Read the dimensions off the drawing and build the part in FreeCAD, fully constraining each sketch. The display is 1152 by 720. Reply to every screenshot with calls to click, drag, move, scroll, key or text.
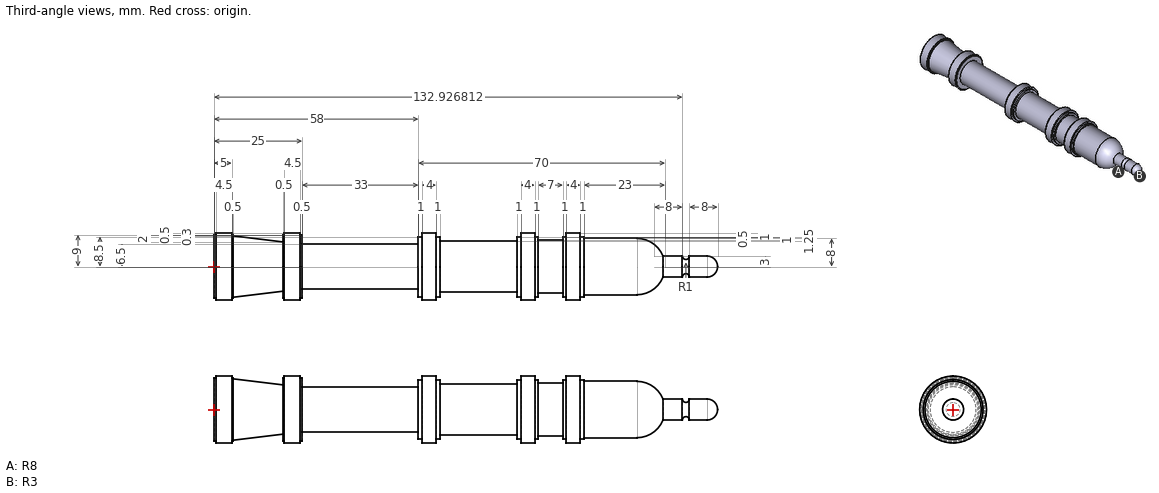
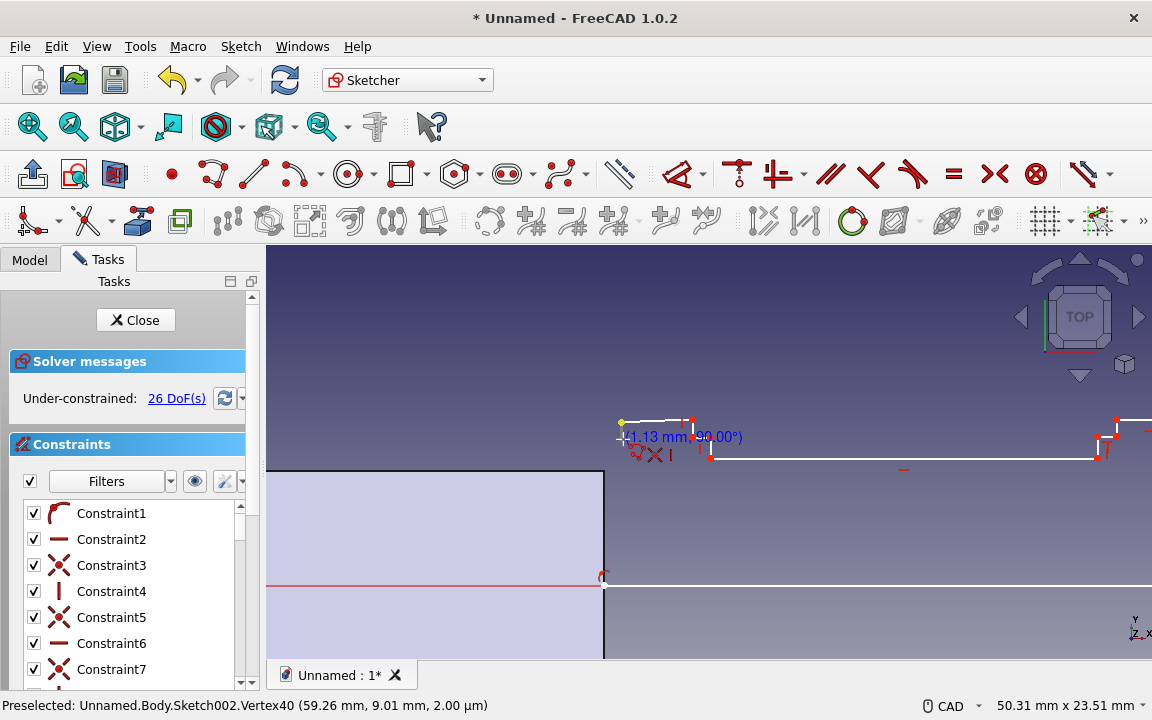
click(621, 436)
click(604, 436)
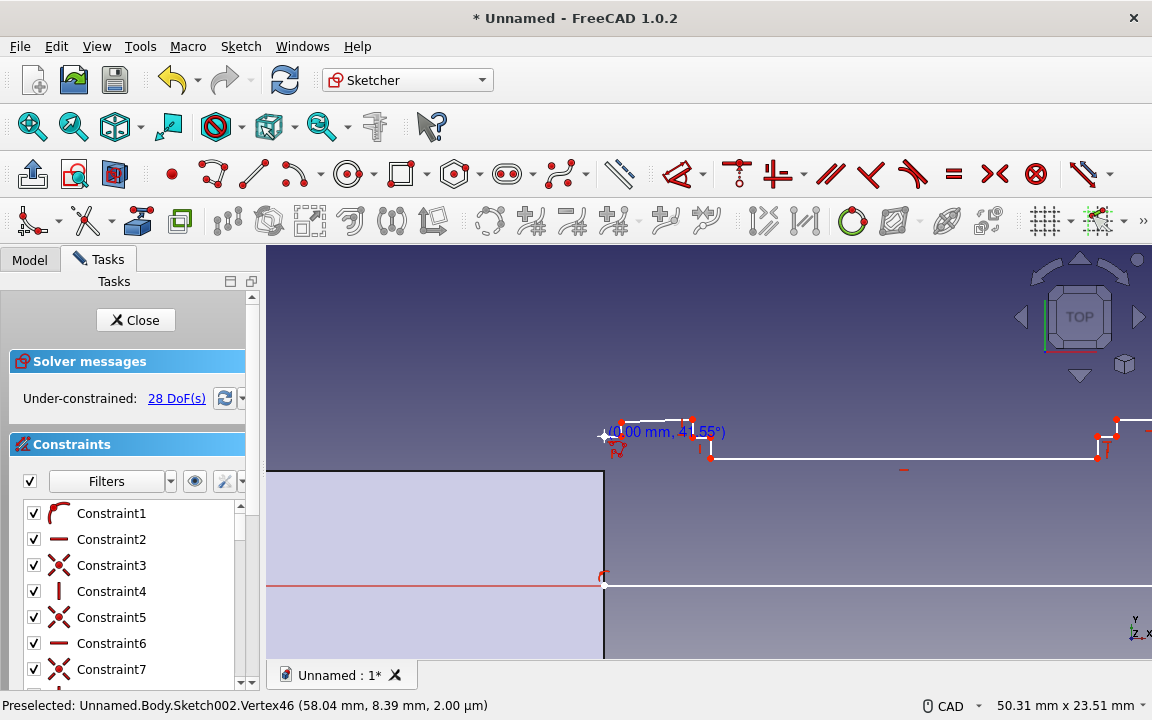
scroll(623, 439, down, 8)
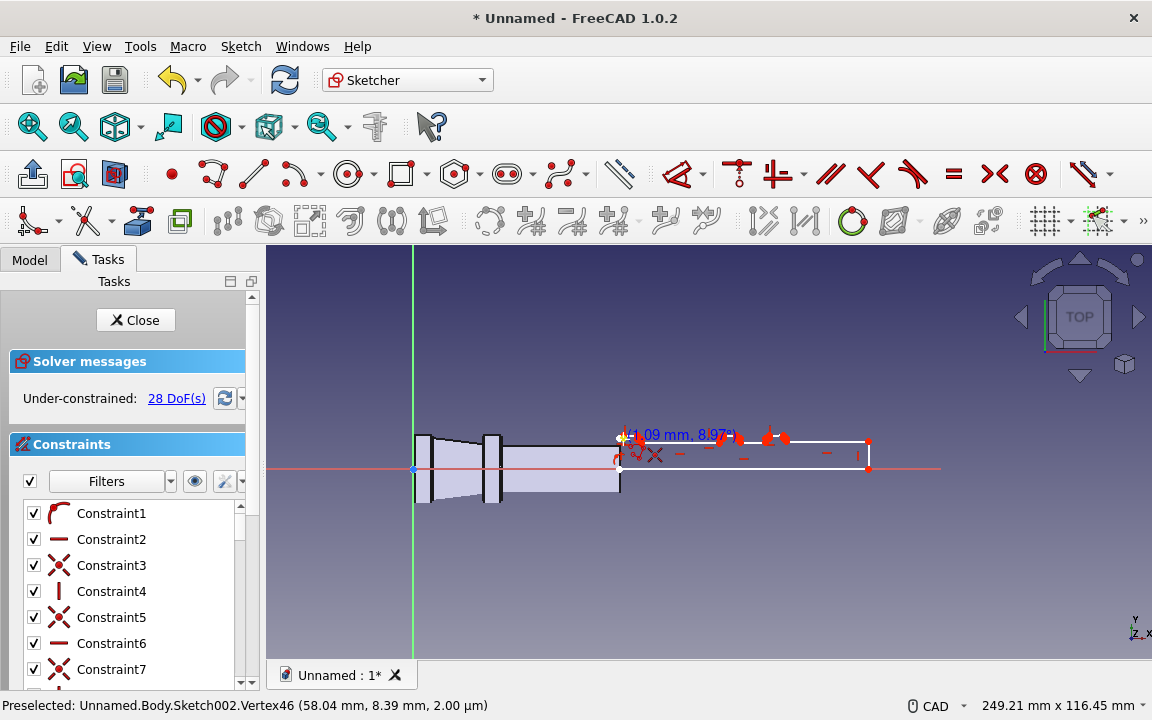
click(620, 469)
key(Escape)
key(Escape)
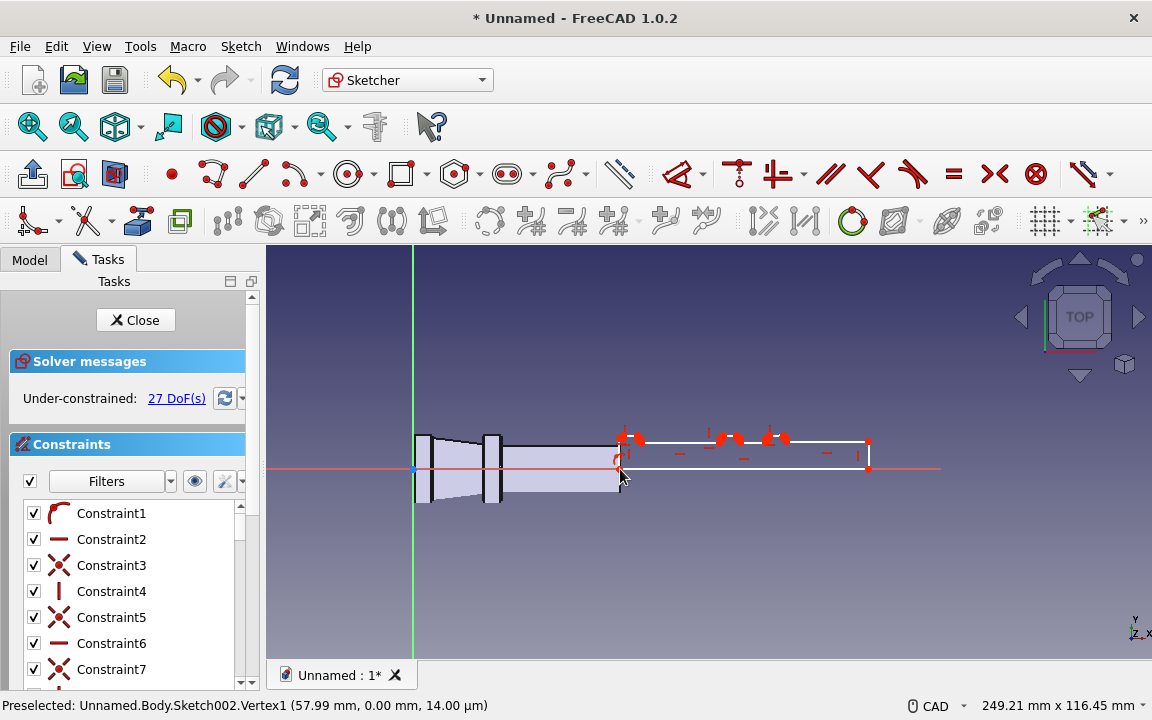
scroll(776, 436, up, 4)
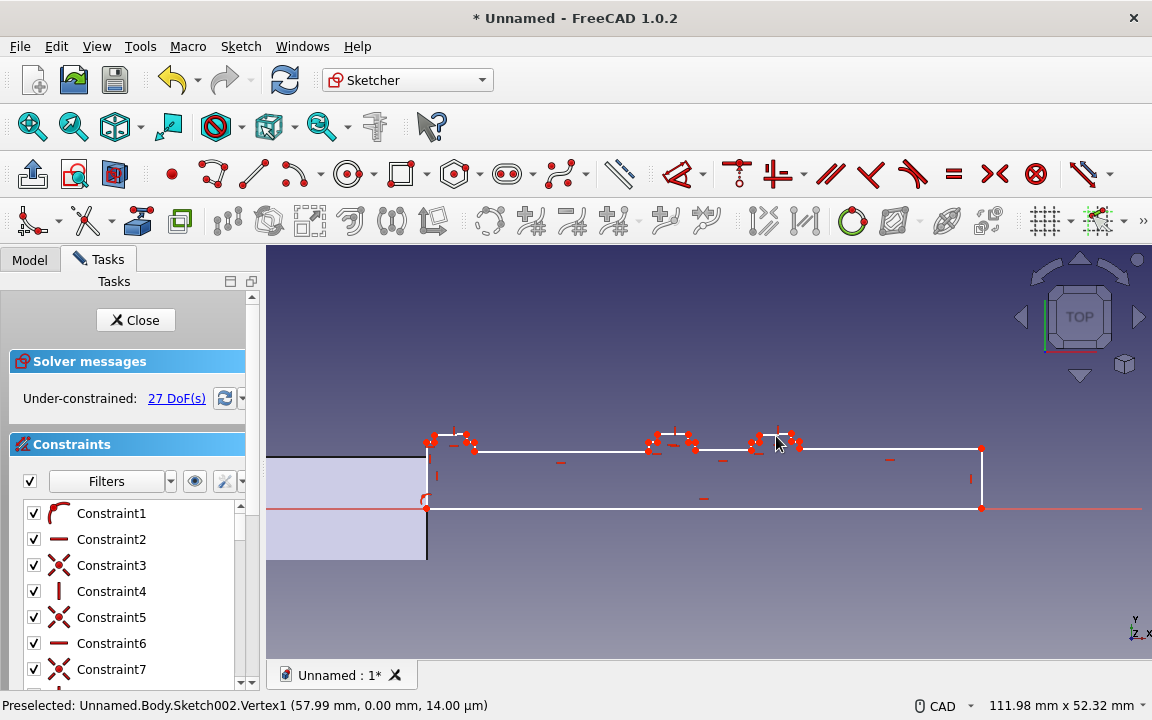
click(772, 435)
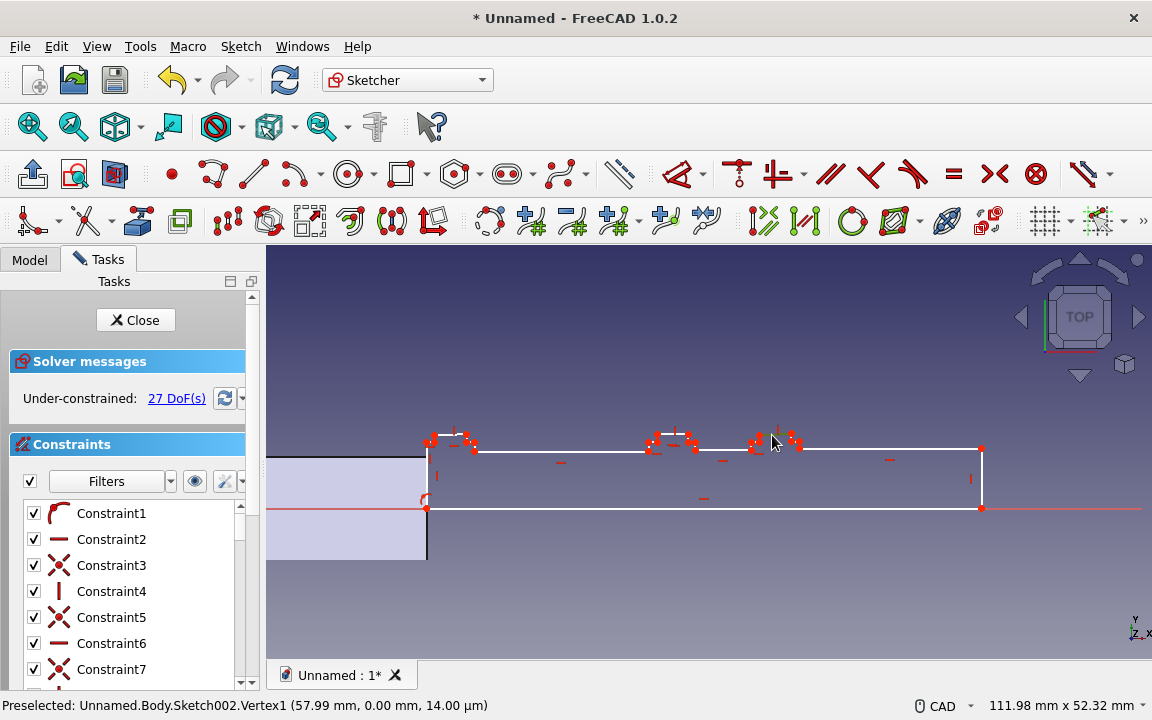
click(804, 174)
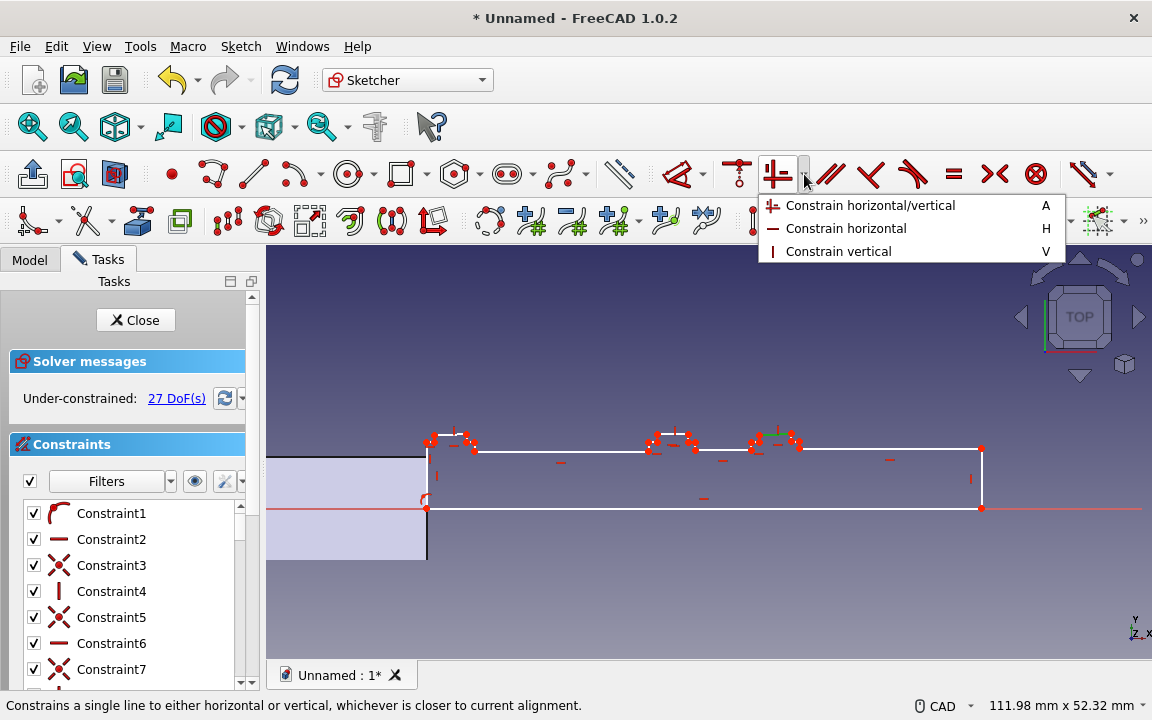
click(912, 228)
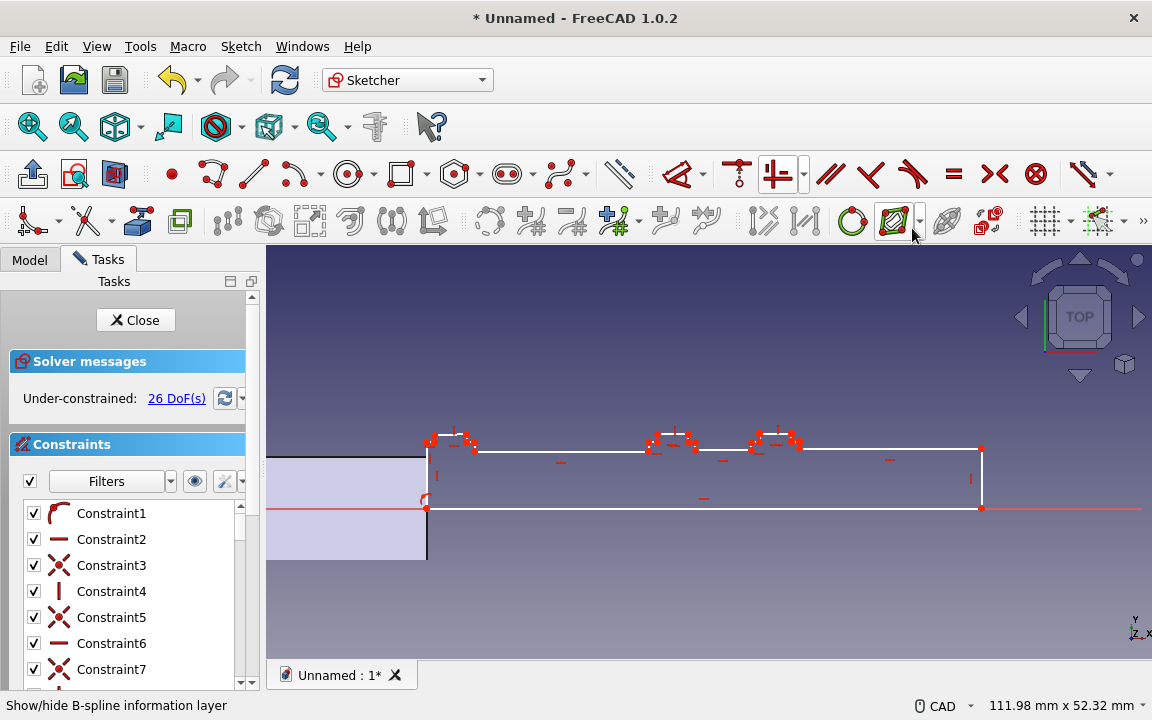
scroll(457, 435, up, 2)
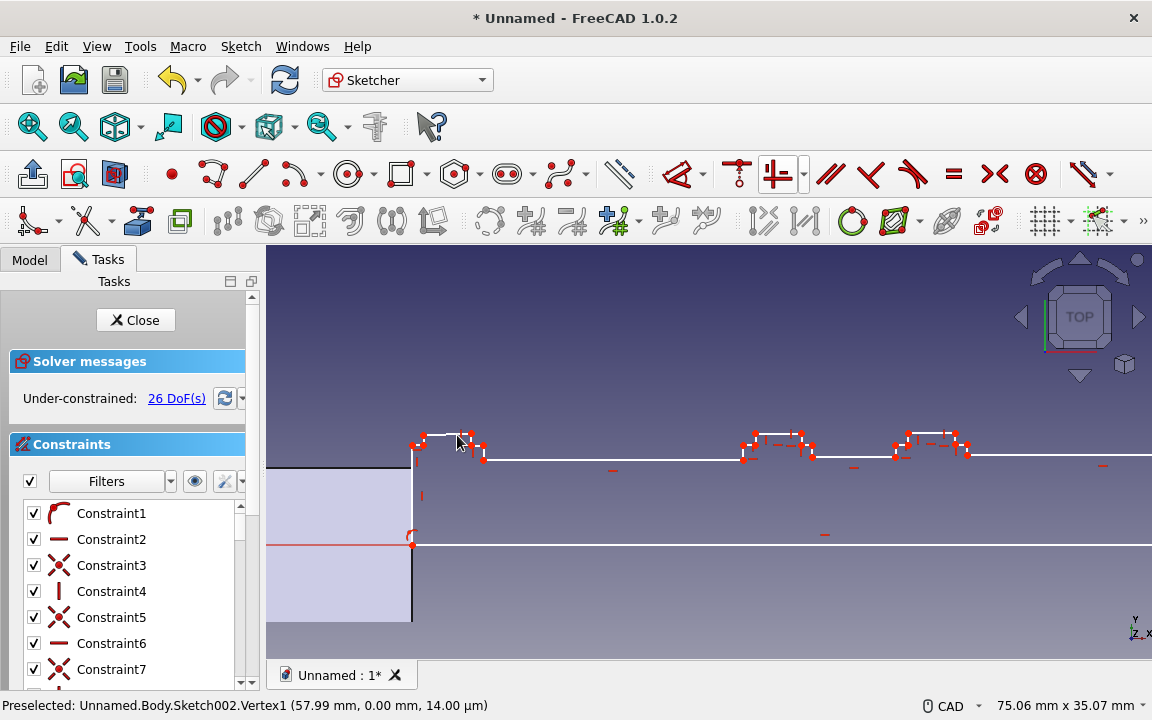
click(438, 435)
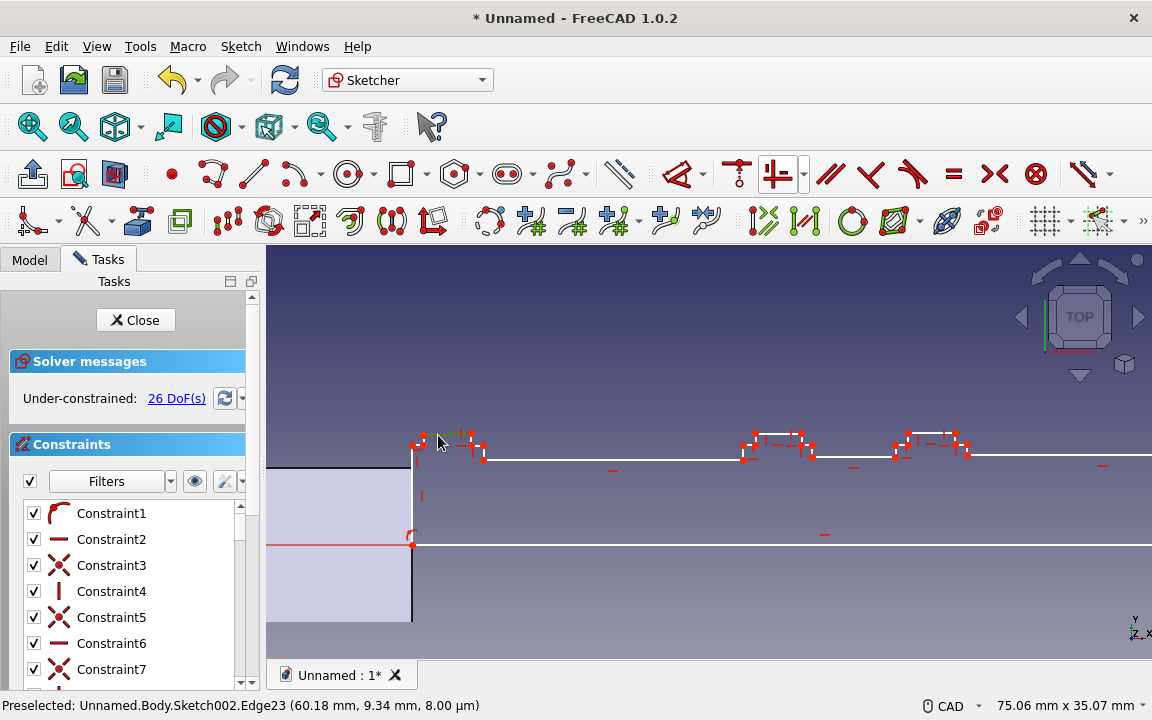
click(804, 174)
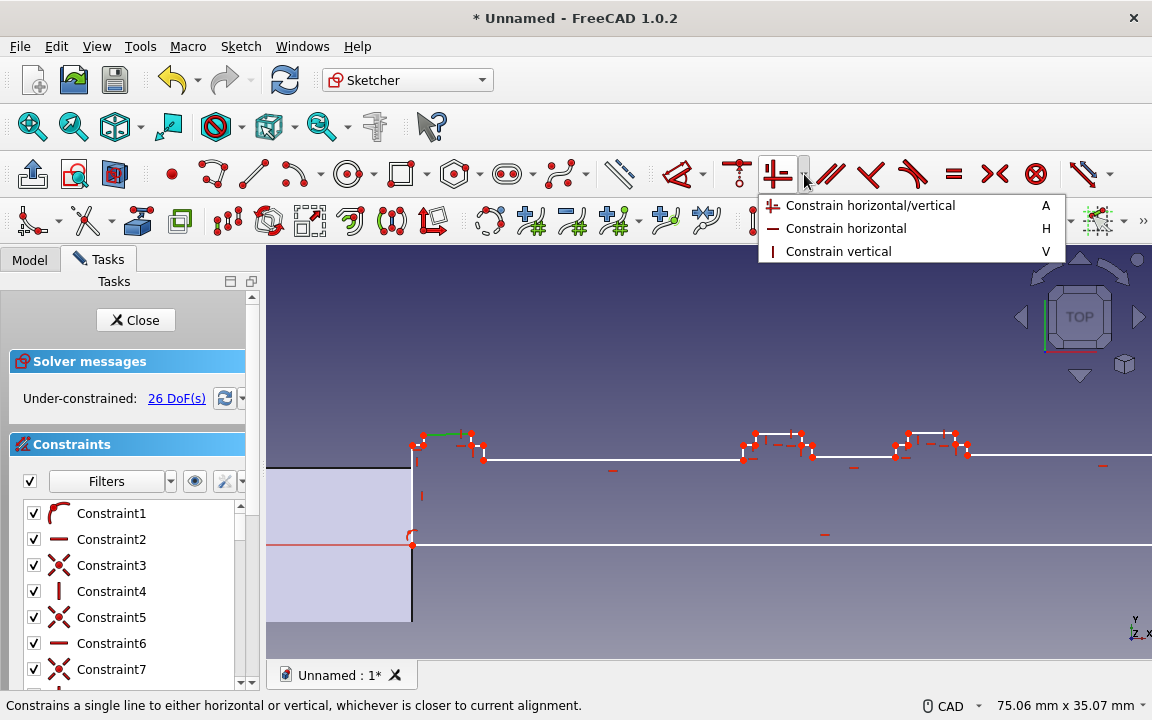
click(912, 228)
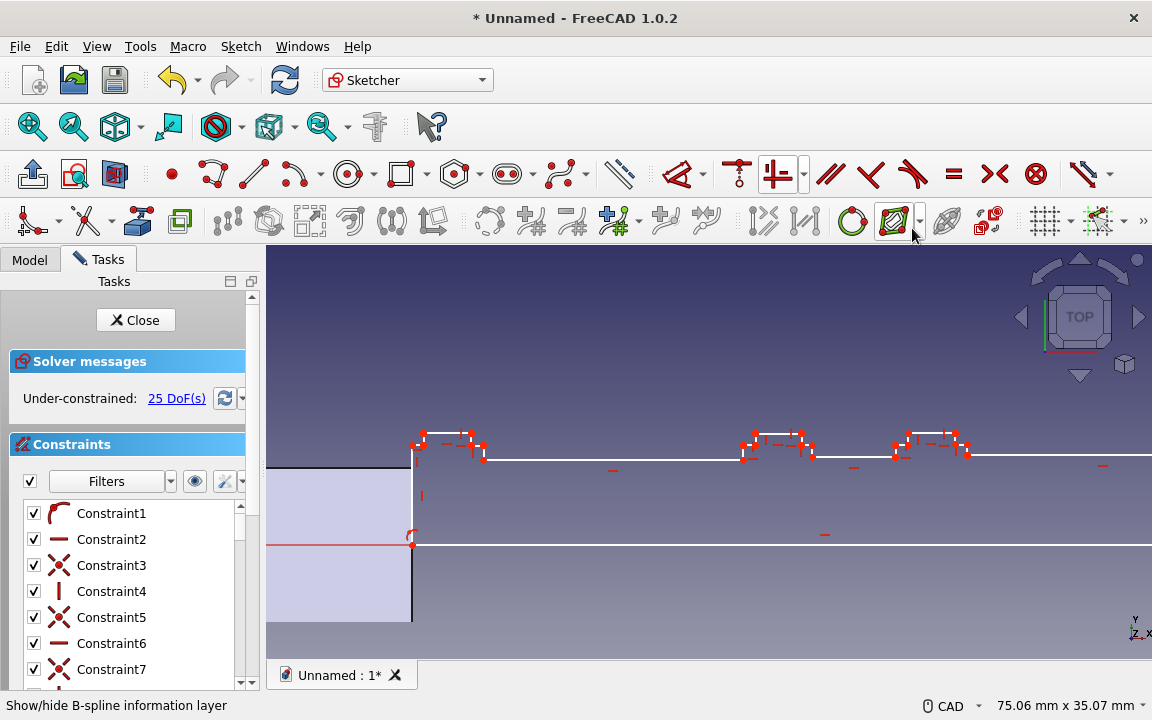
click(676, 174)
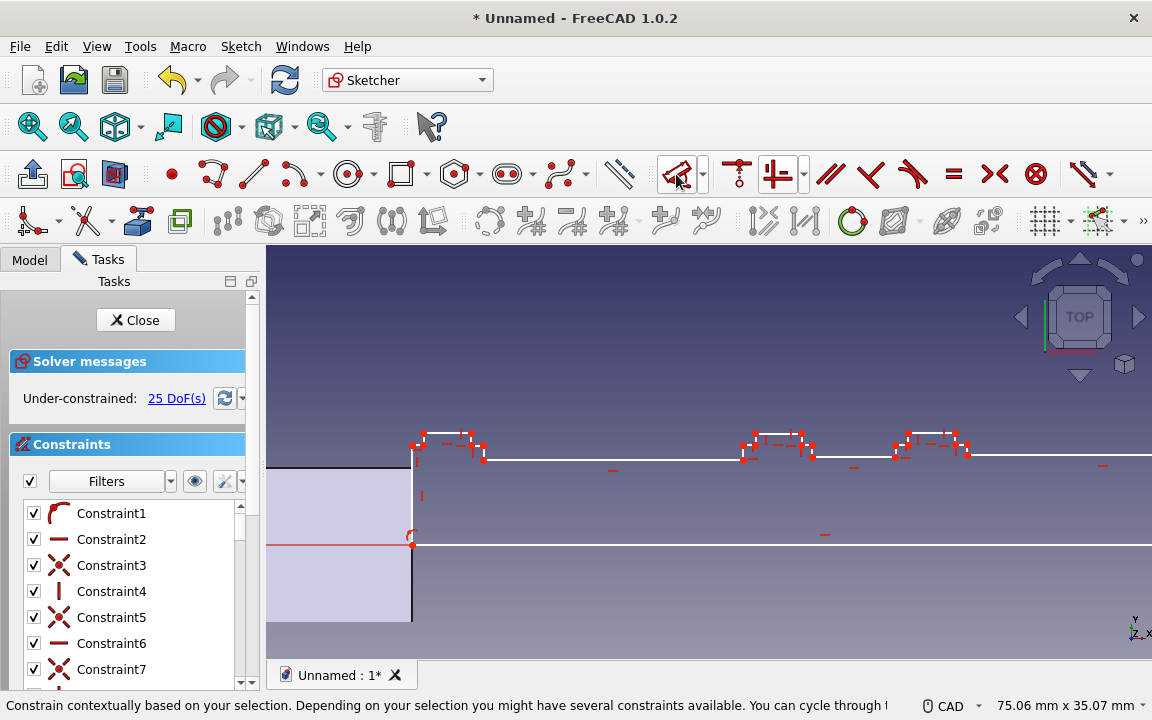
scroll(708, 436, down, 6)